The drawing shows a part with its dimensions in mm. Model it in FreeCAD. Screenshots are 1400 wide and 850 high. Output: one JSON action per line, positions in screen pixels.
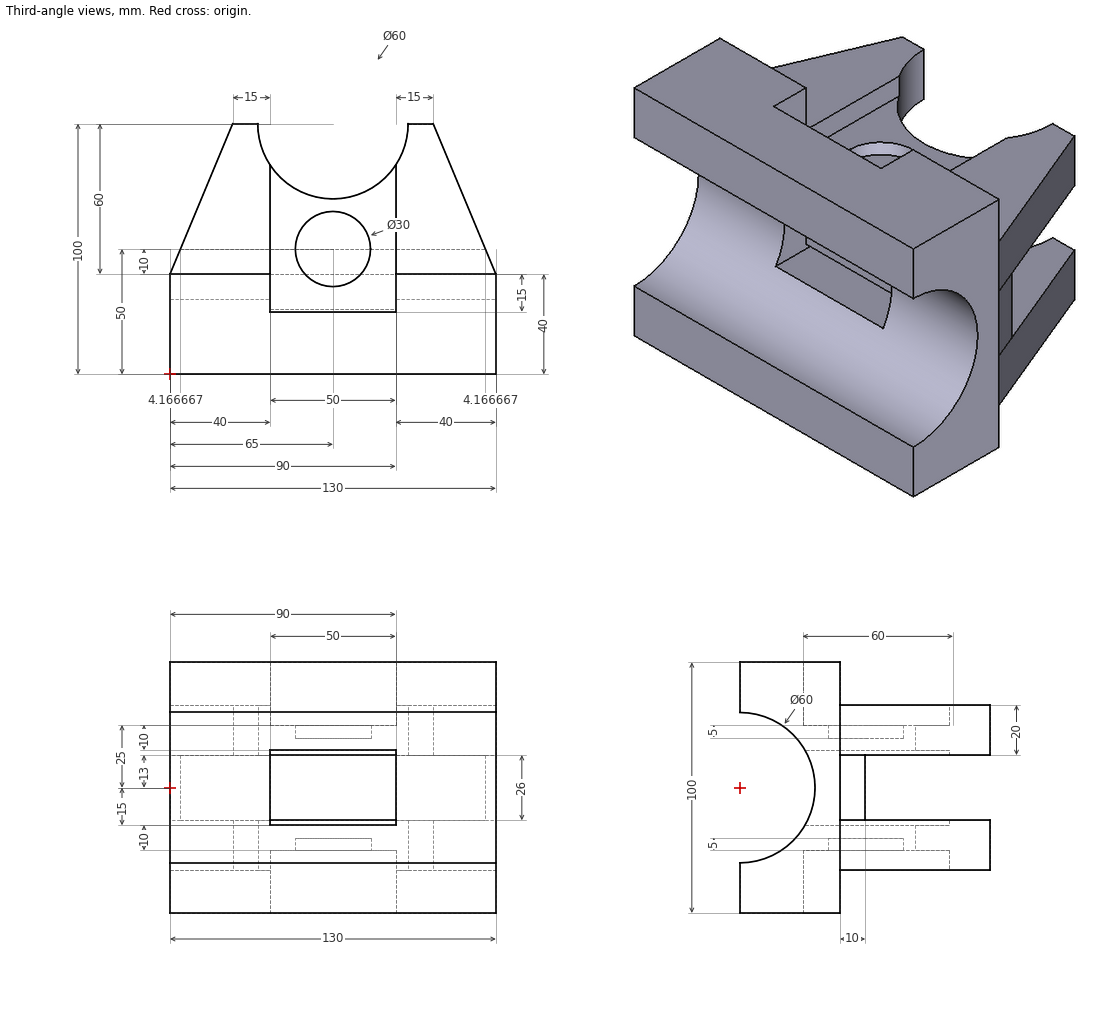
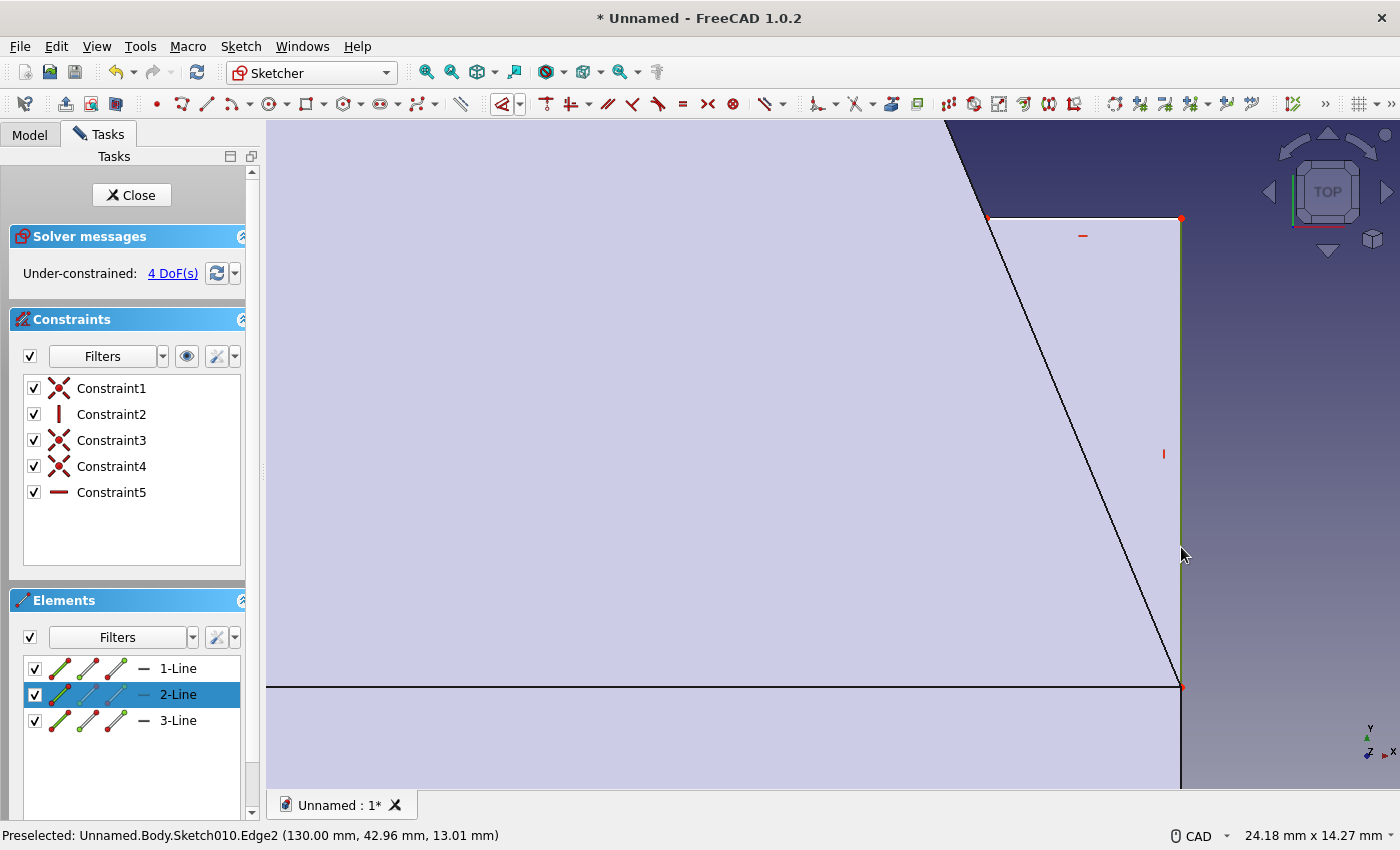
{"action": "left_click", "coordinate": [520, 104]}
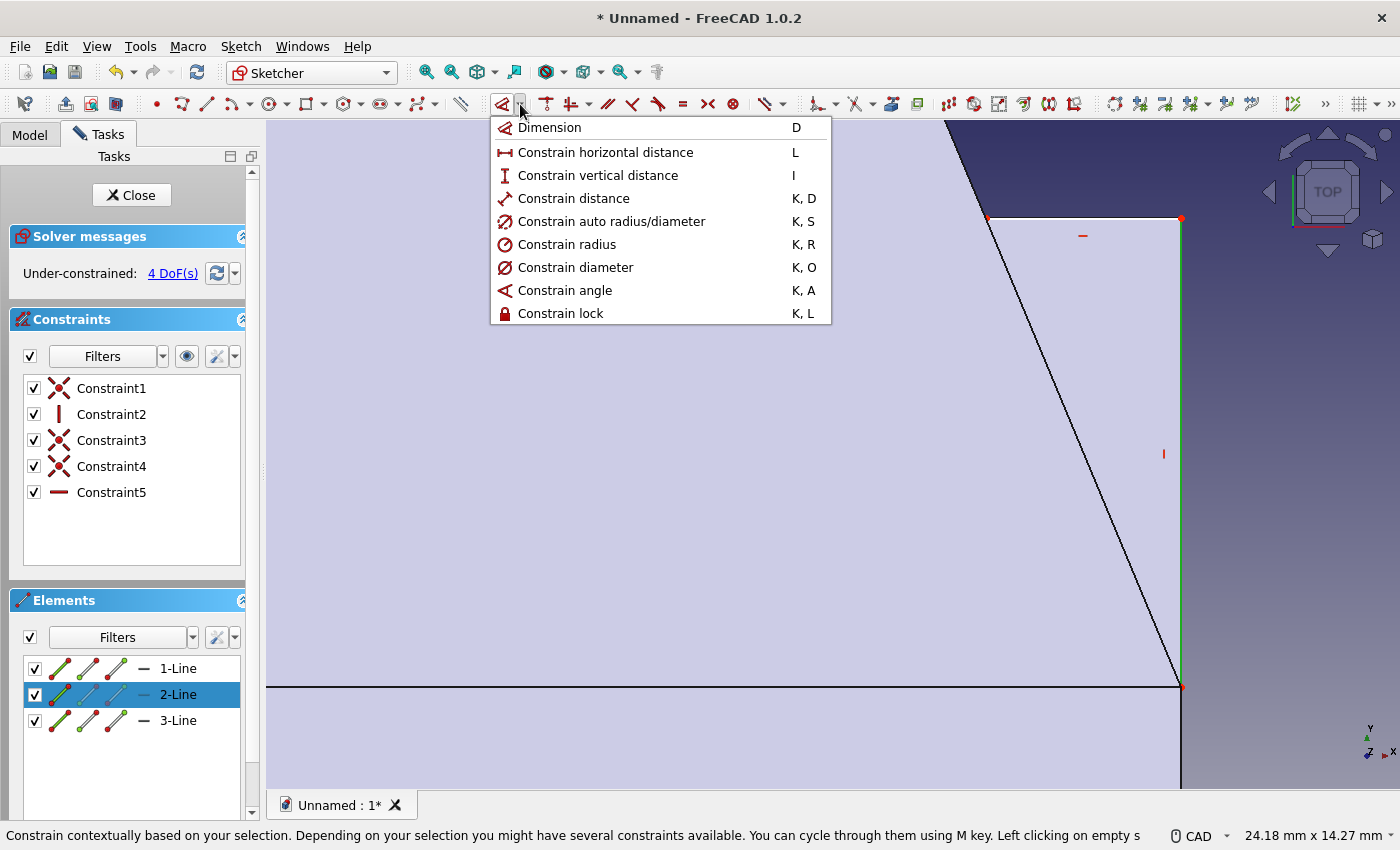
{"action": "left_click", "coordinate": [661, 176]}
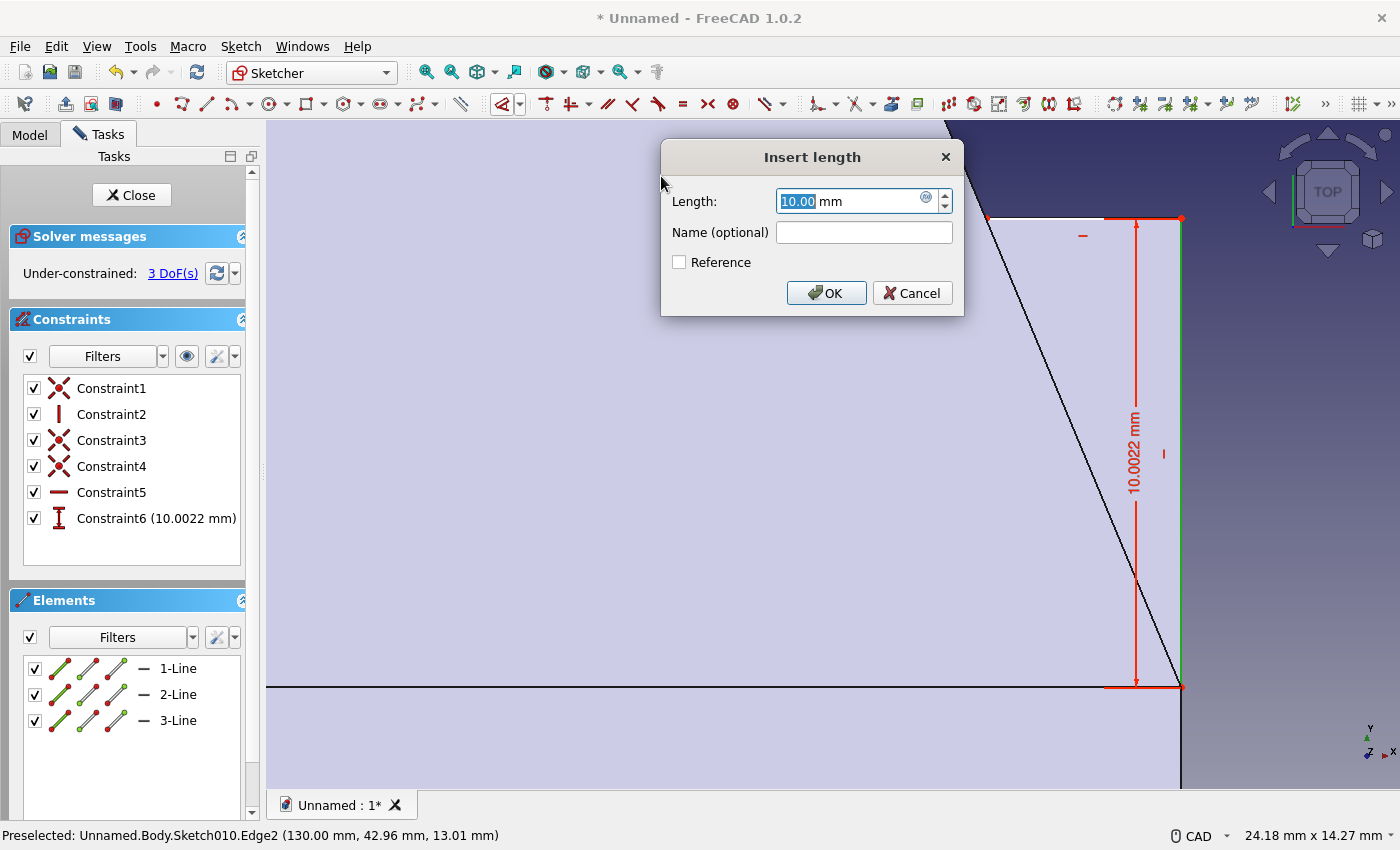
{"action": "type", "text": "10"}
{"action": "key", "text": "Return"}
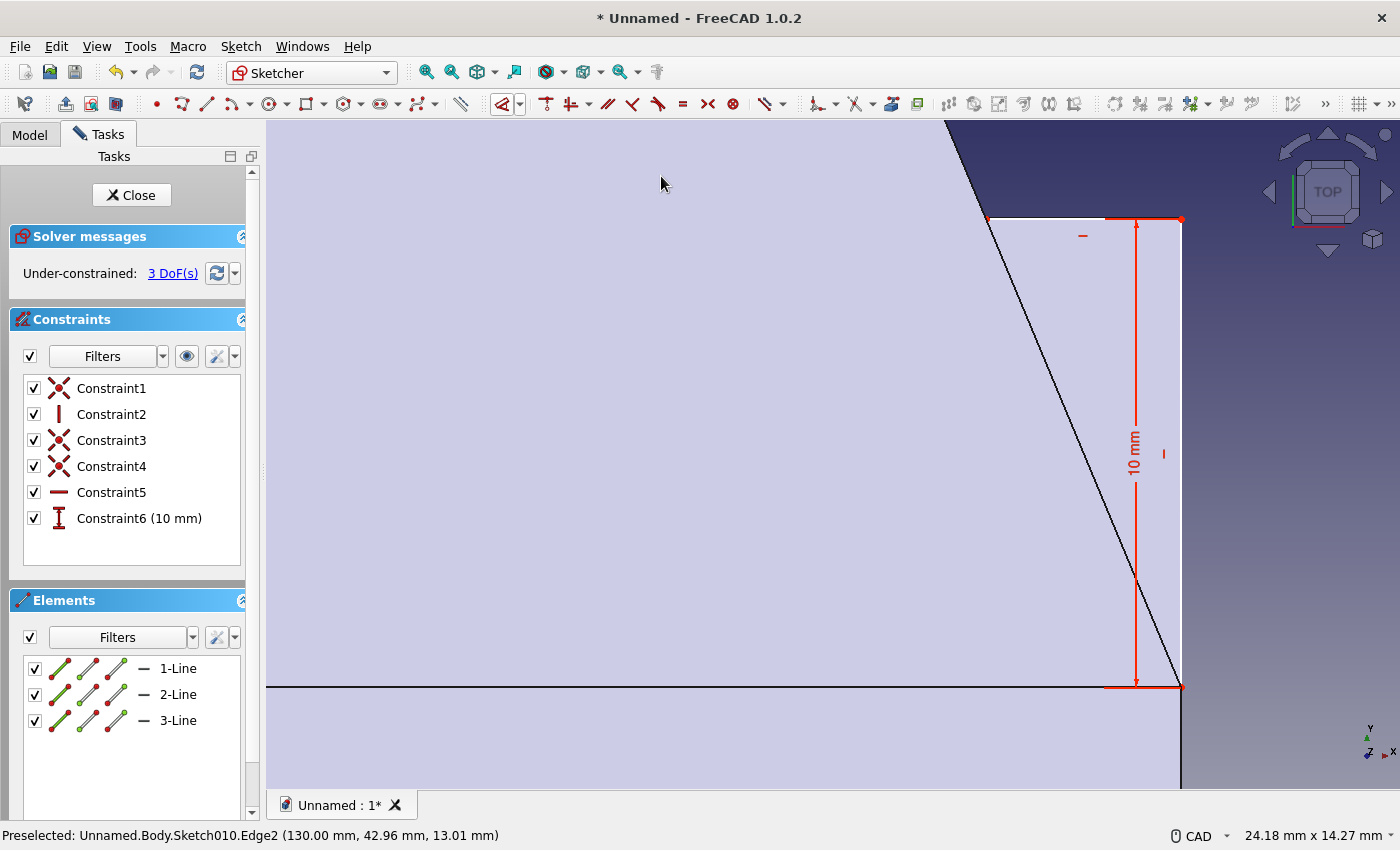
{"action": "left_click", "coordinate": [986, 219]}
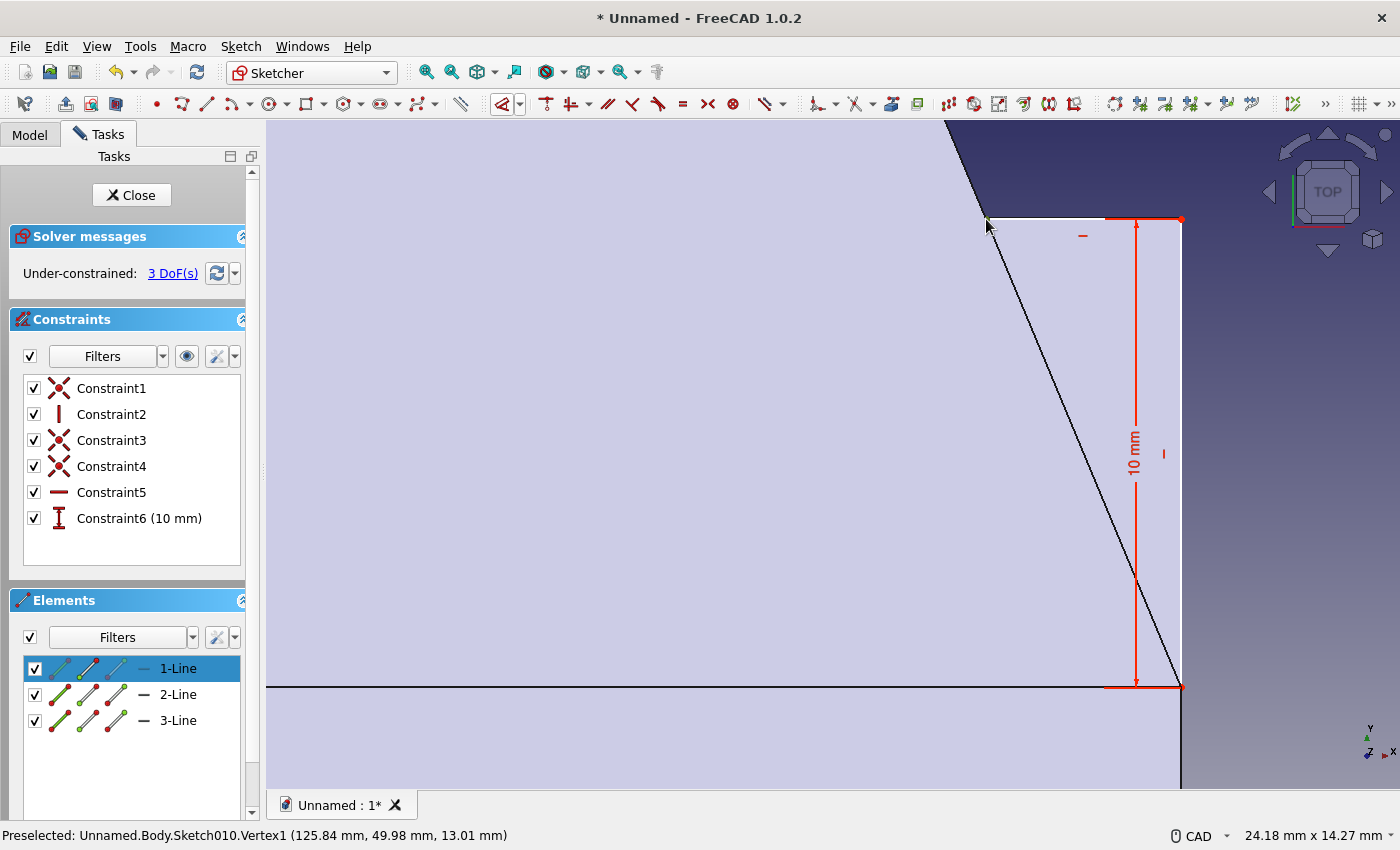
{"action": "left_click", "coordinate": [520, 104]}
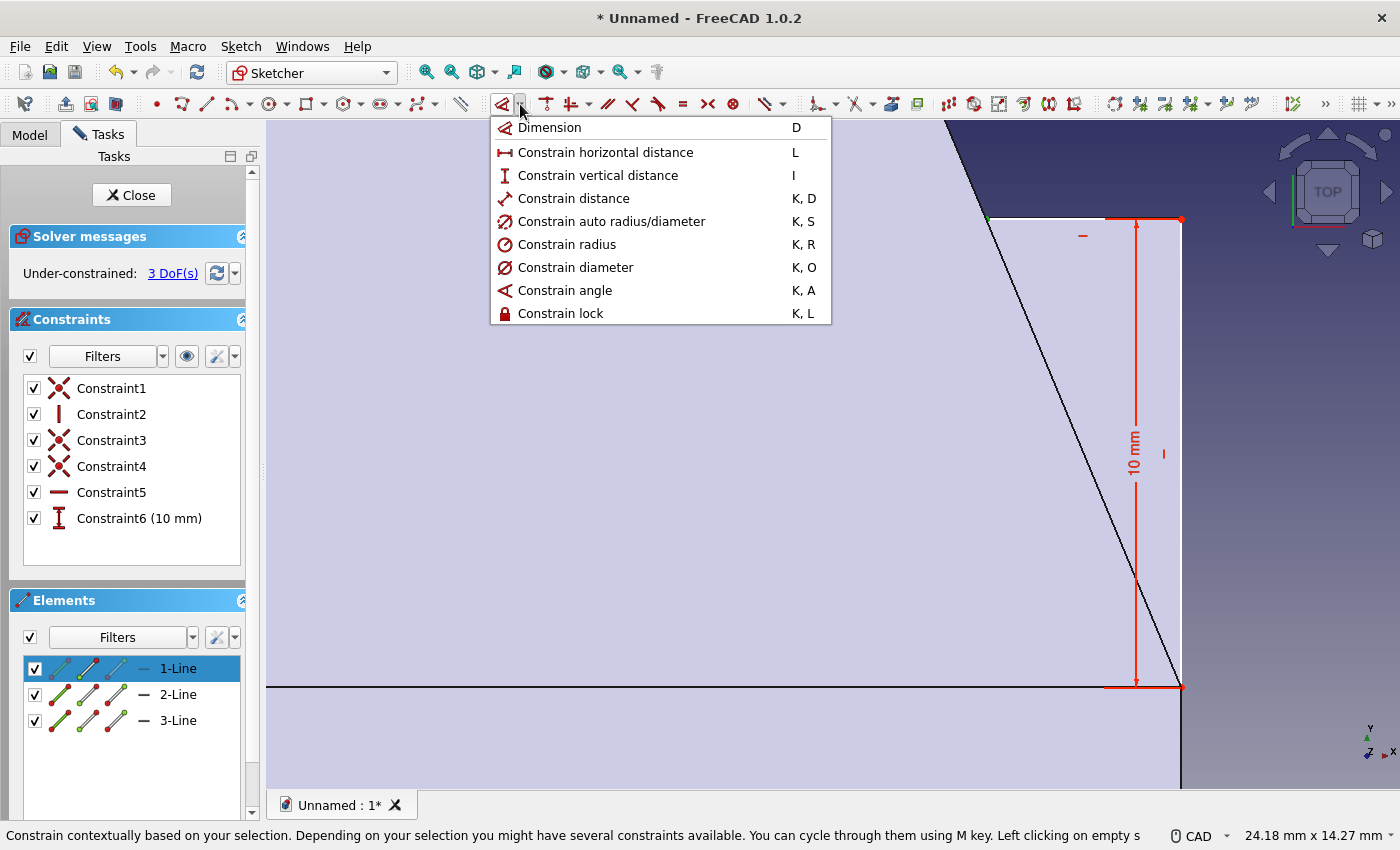
{"action": "left_click", "coordinate": [661, 176]}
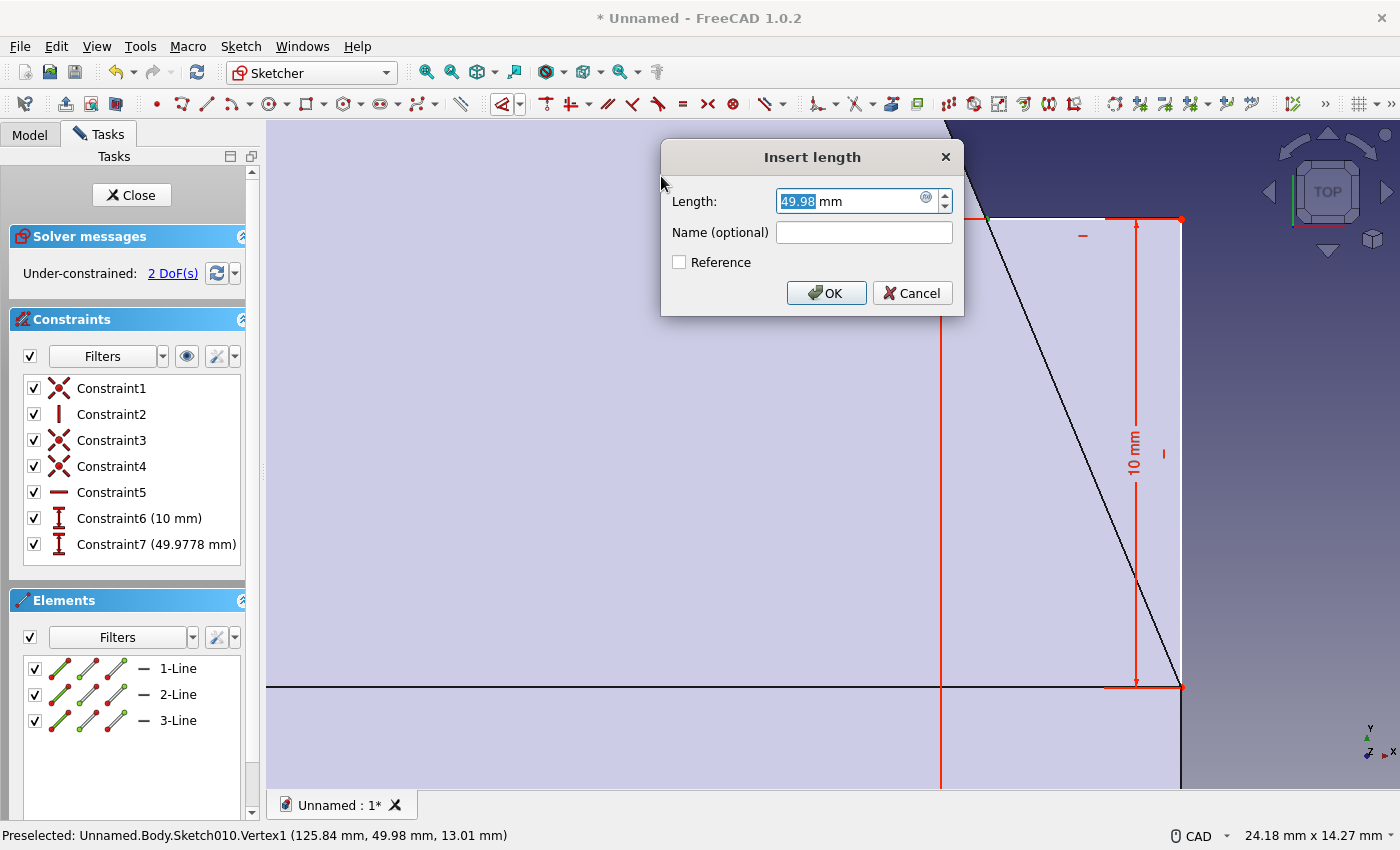
{"action": "type", "text": "50"}
{"action": "key", "text": "Return"}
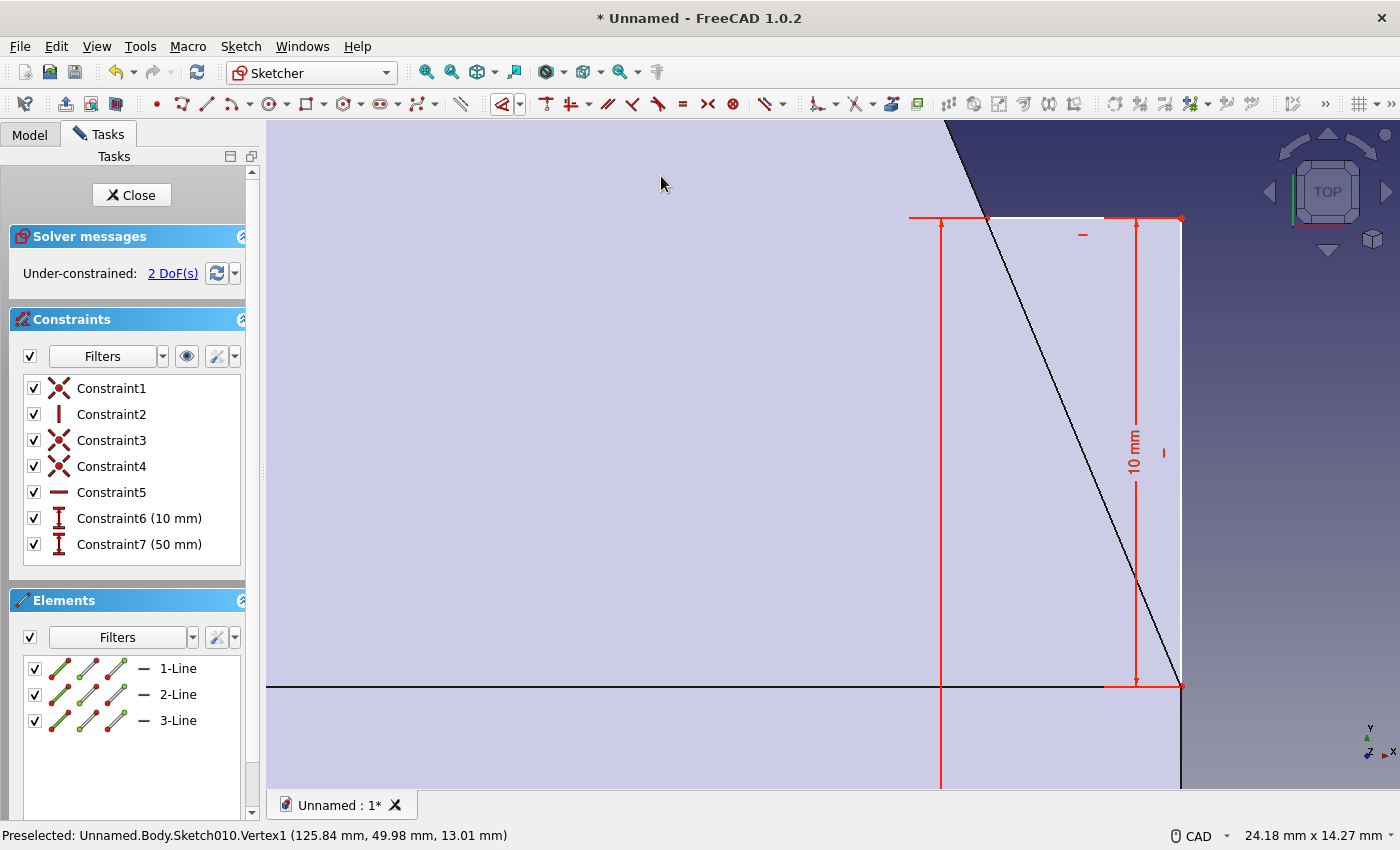
{"action": "left_click", "coordinate": [1181, 687]}